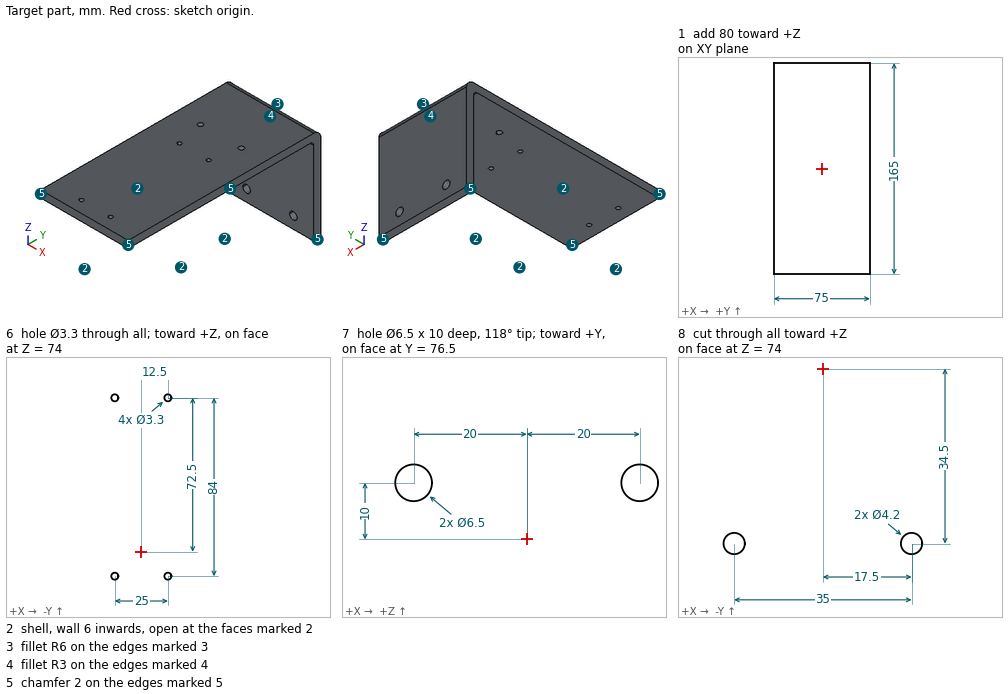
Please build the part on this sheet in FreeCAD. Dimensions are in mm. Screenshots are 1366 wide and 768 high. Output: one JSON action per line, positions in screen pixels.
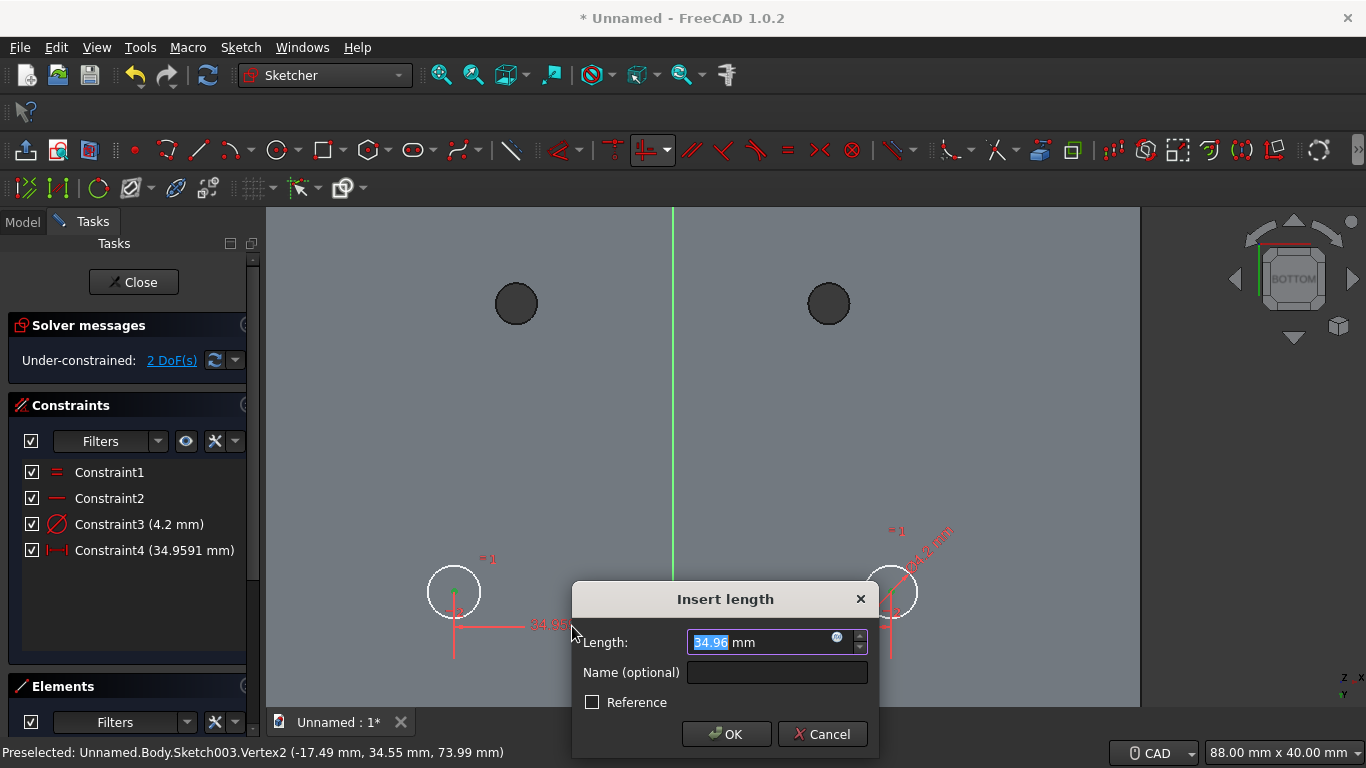
{"action": "type", "text": "35"}
{"action": "key", "text": "Return"}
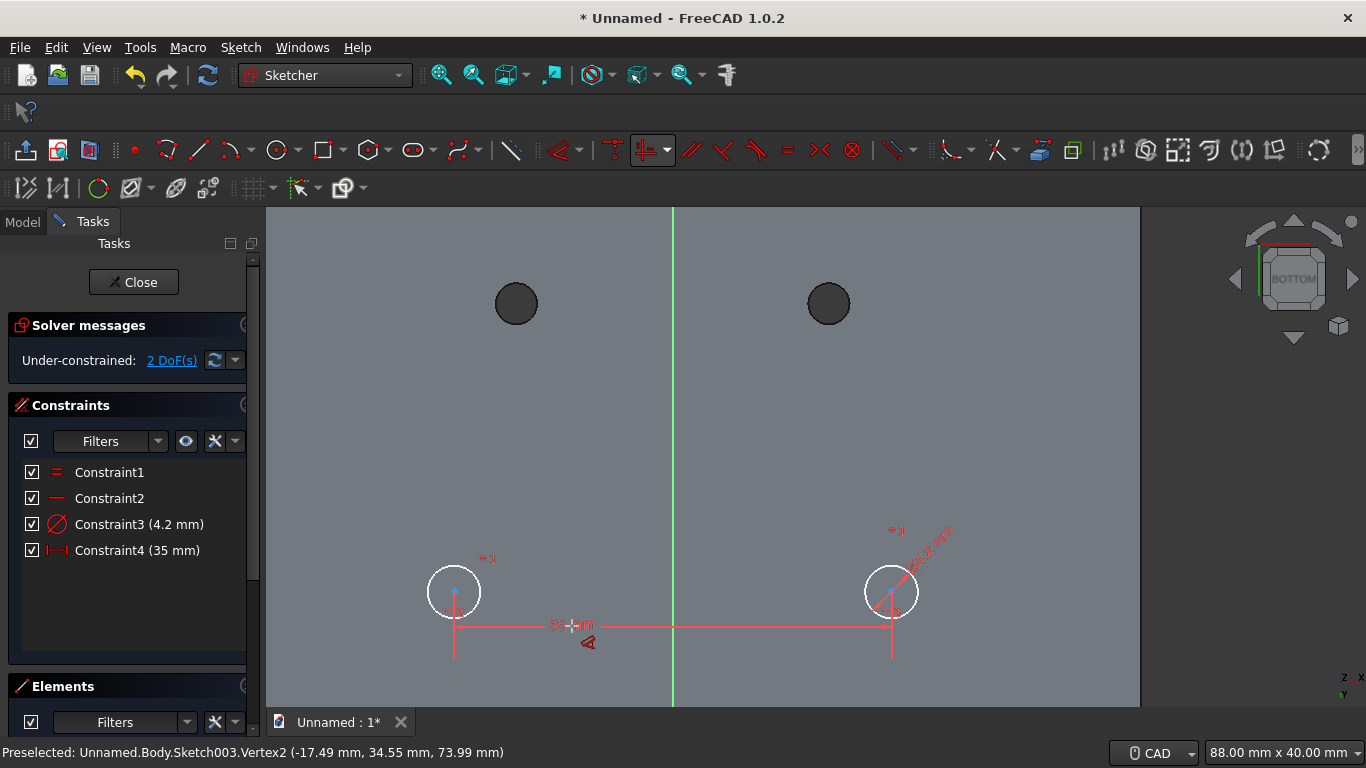
{"action": "left_click", "coordinate": [892, 592]}
{"action": "left_click", "coordinate": [782, 626]}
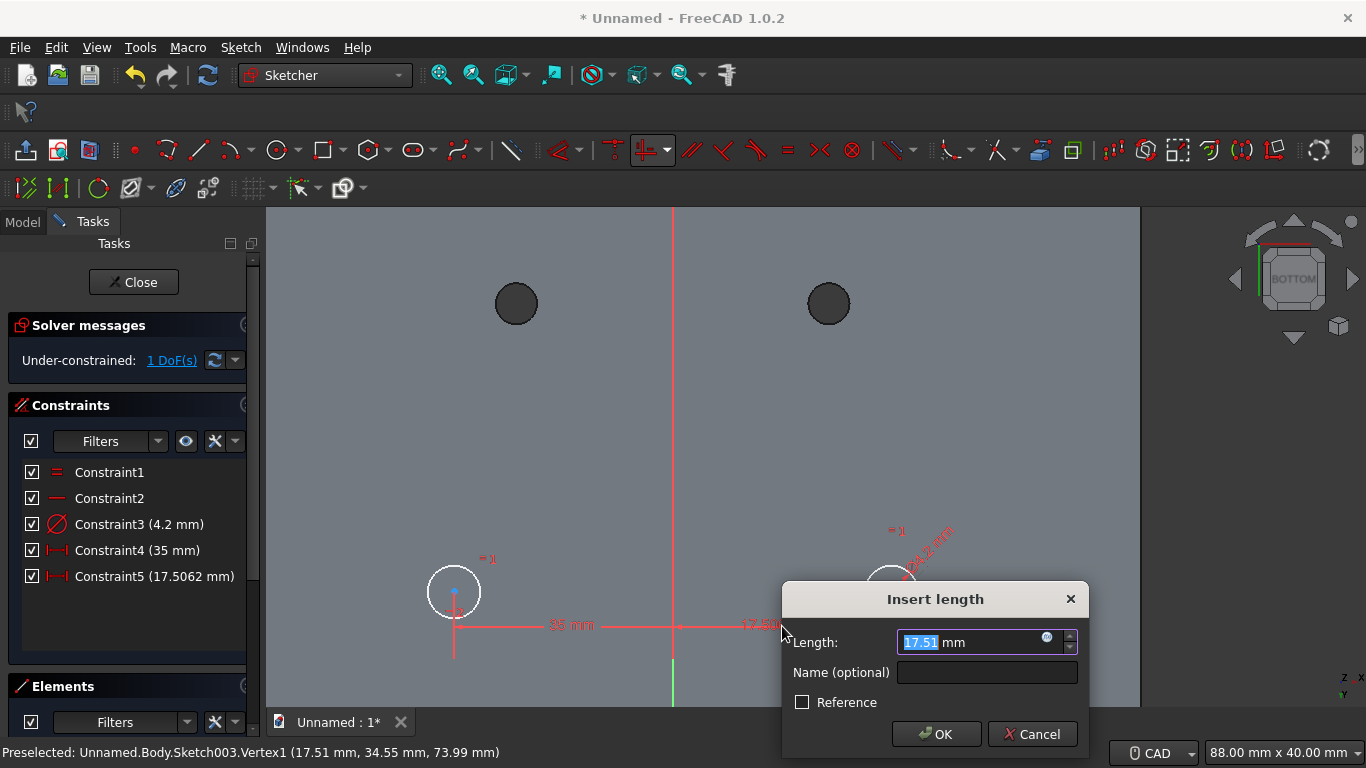
{"action": "type", "text": "17.5"}
{"action": "key", "text": "Return"}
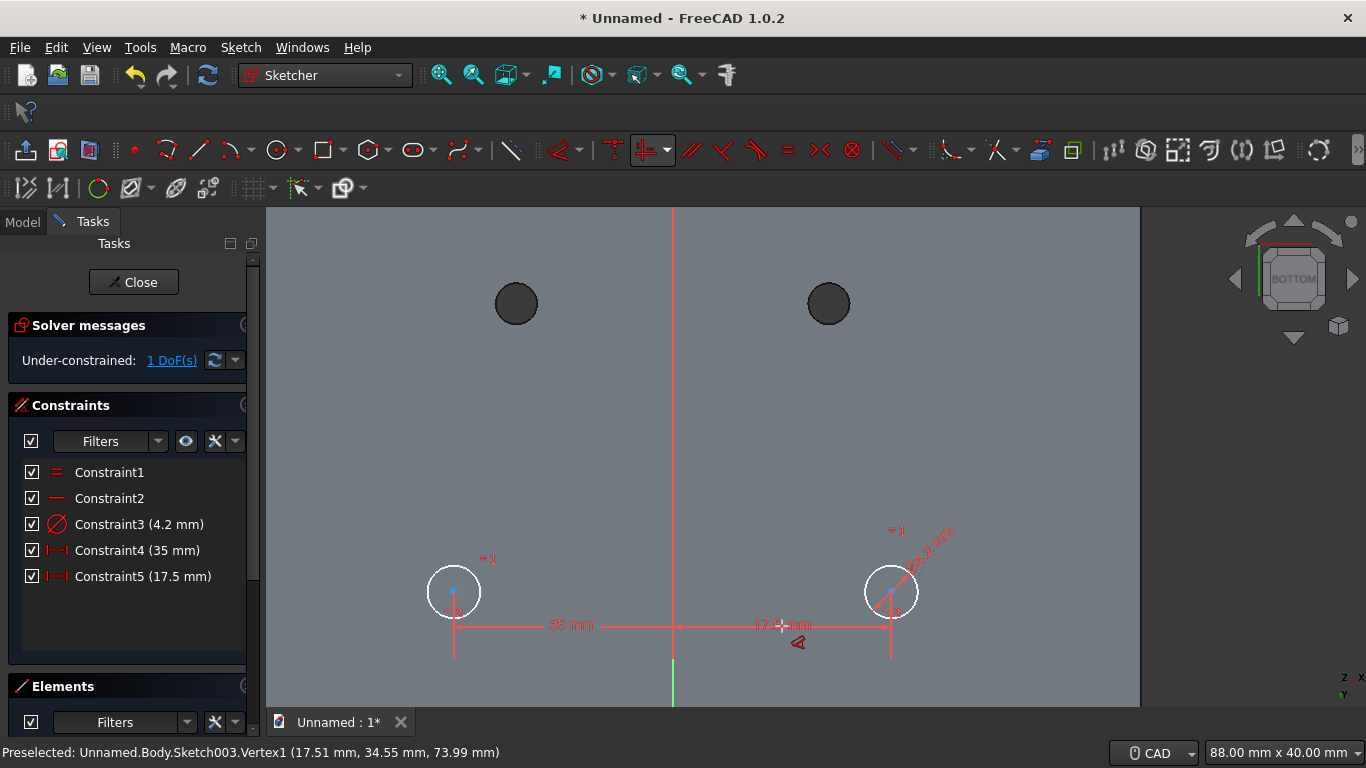
{"action": "left_click", "coordinate": [891, 592]}
{"action": "left_click", "coordinate": [925, 414]}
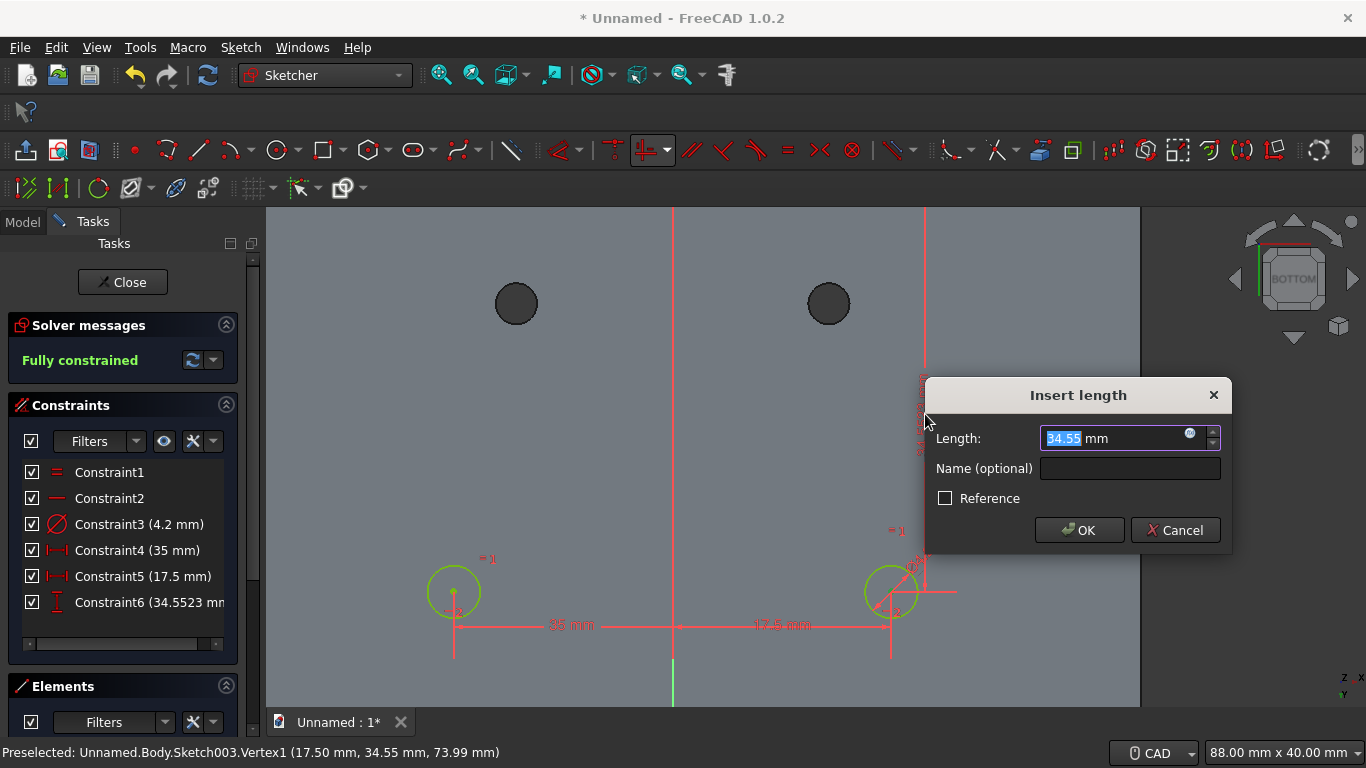
{"action": "type", "text": "34.5"}
{"action": "key", "text": "Return"}
{"action": "key", "text": "Escape"}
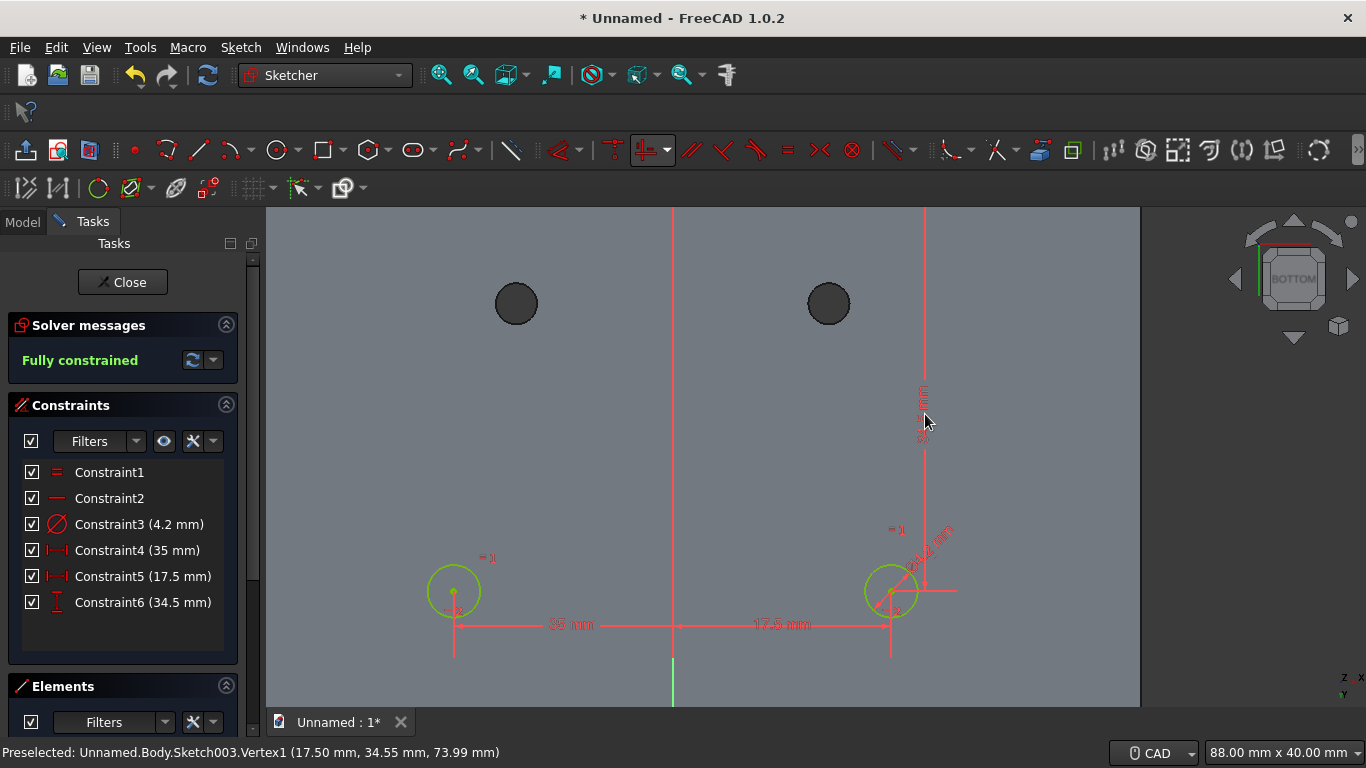
{"action": "left_click", "coordinate": [123, 282]}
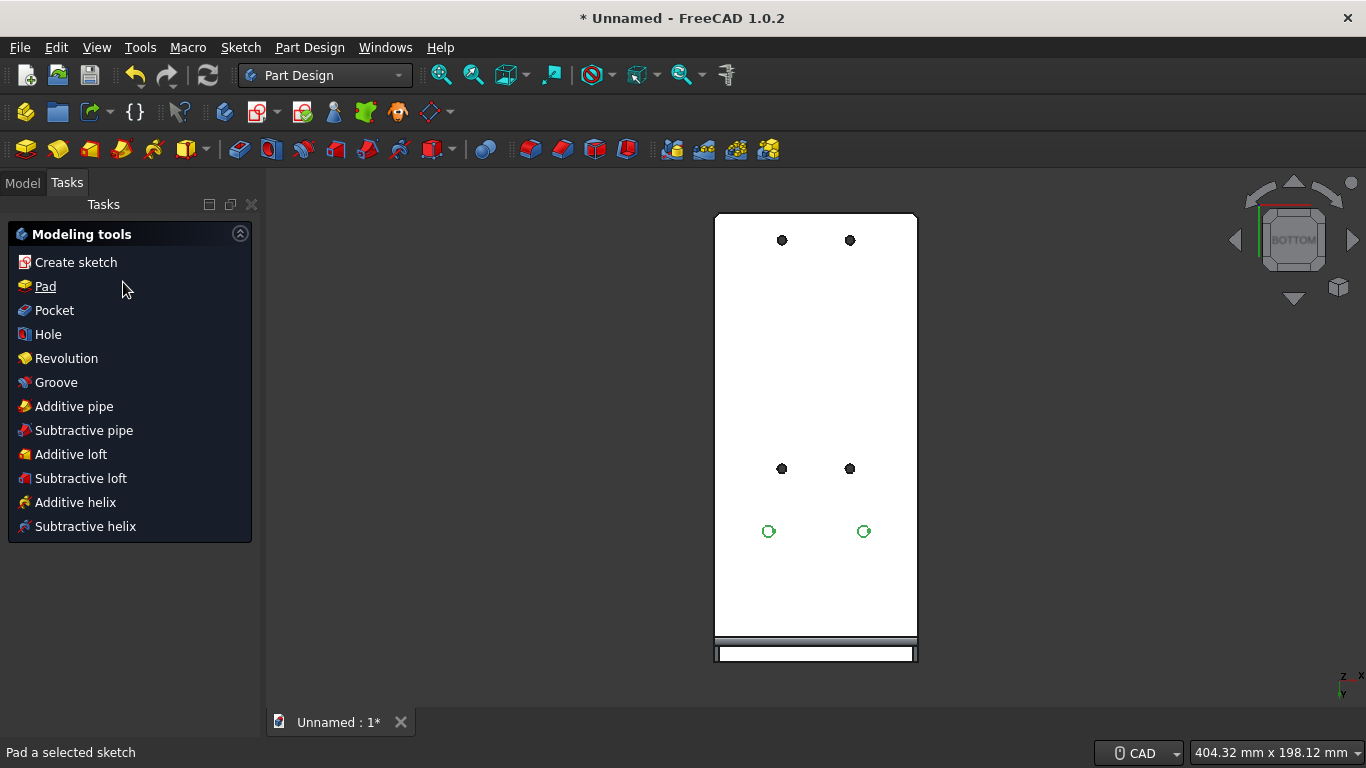
{"action": "left_click", "coordinate": [240, 150]}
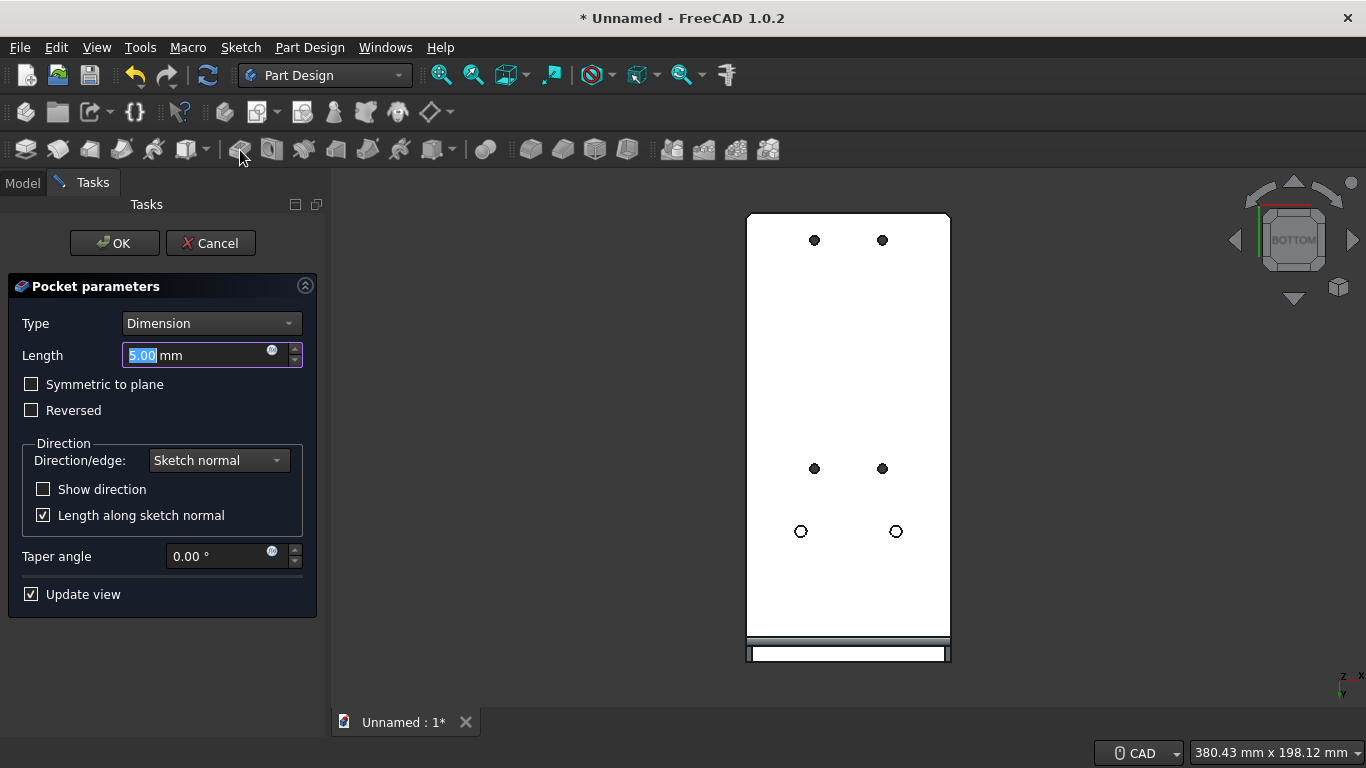
{"action": "left_click", "coordinate": [212, 324]}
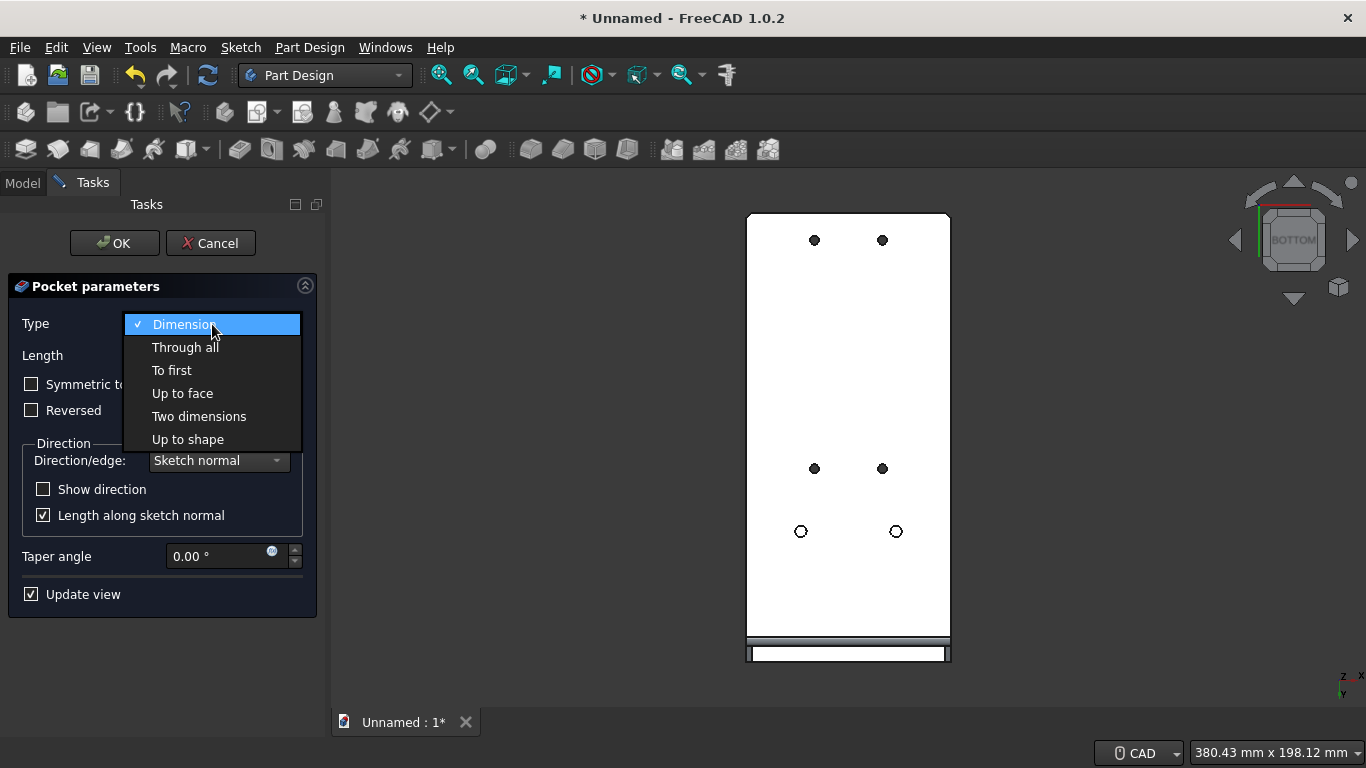
{"action": "left_click", "coordinate": [212, 348]}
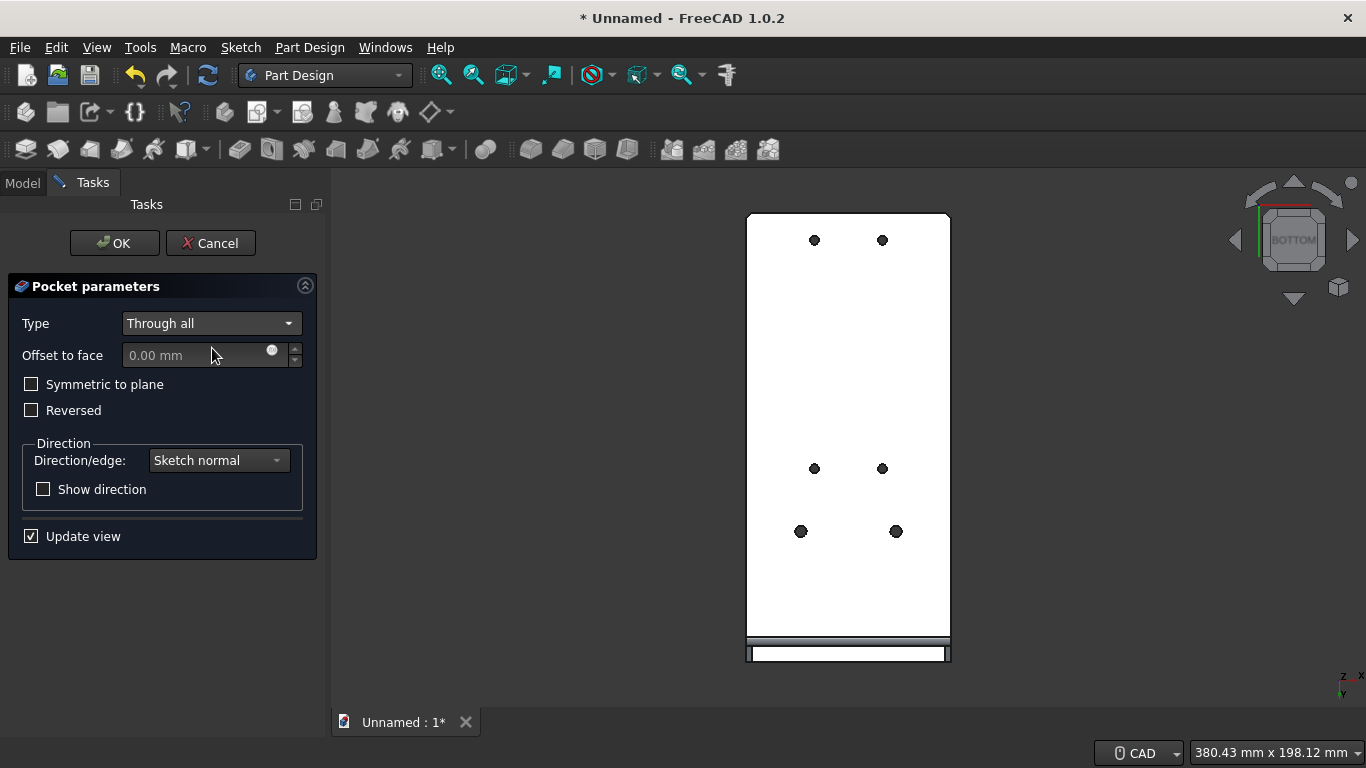
{"action": "left_click", "coordinate": [115, 243]}